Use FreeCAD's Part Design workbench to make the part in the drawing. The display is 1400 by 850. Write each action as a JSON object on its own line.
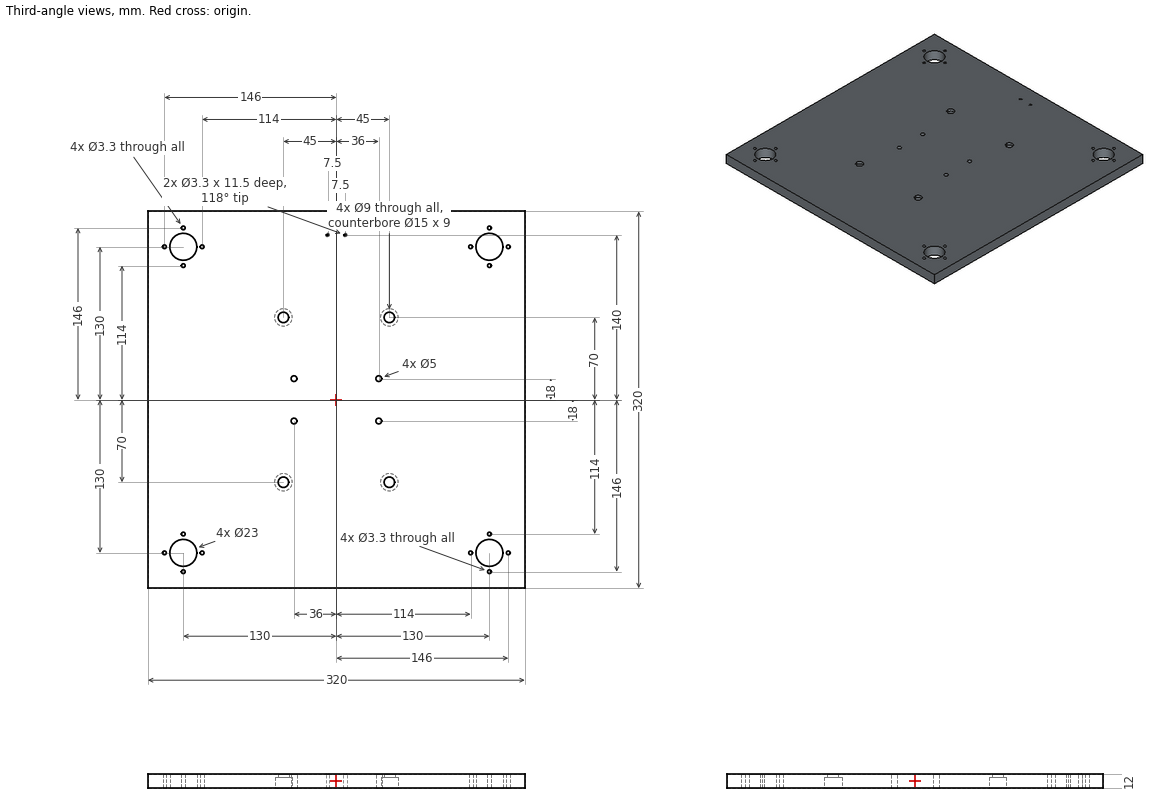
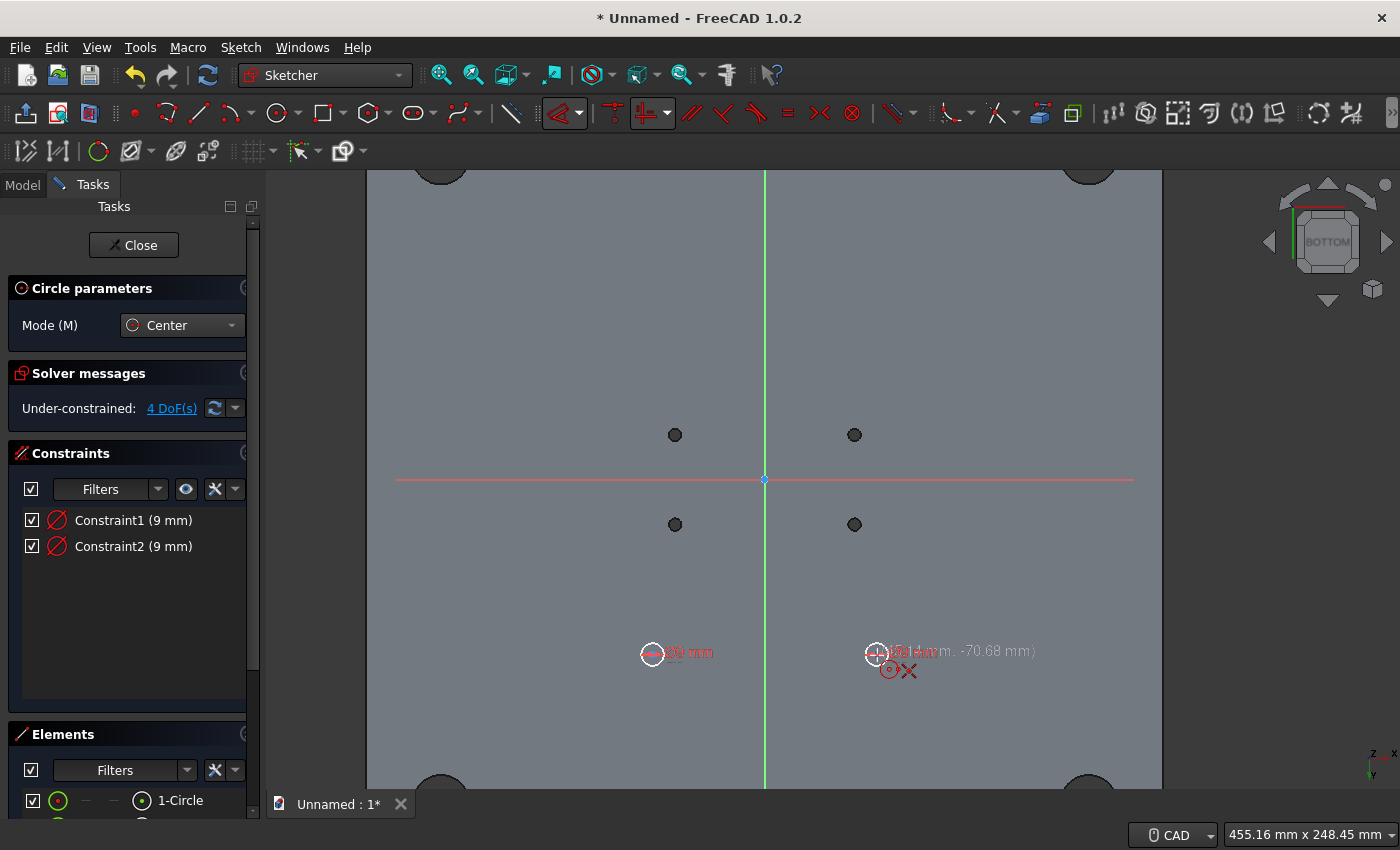
{"action": "scroll", "coordinate": [653, 305], "scroll_direction": "up", "scroll_amount": 4}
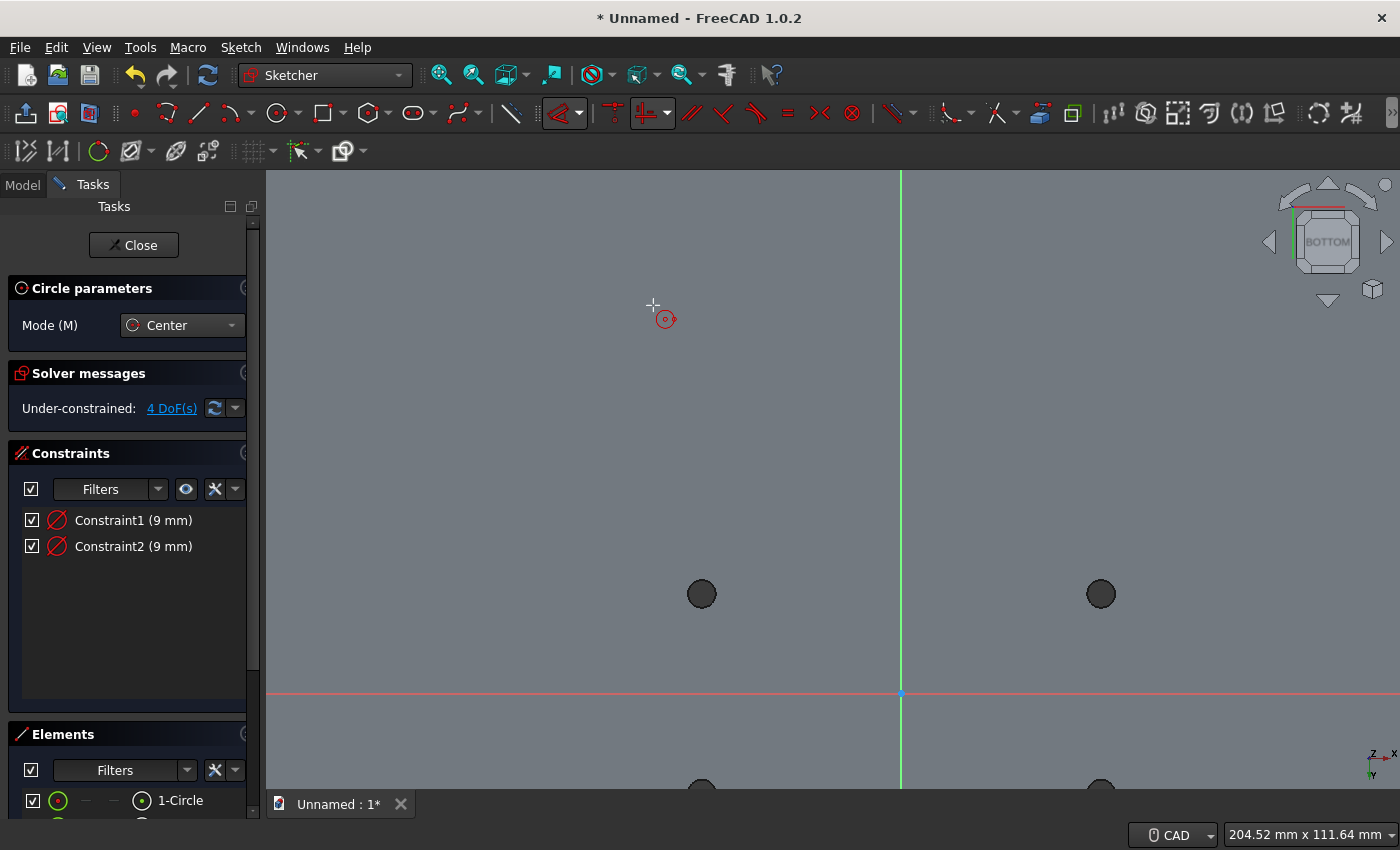
{"action": "left_click", "coordinate": [652, 306]}
{"action": "mouse_move", "coordinate": [670, 288]}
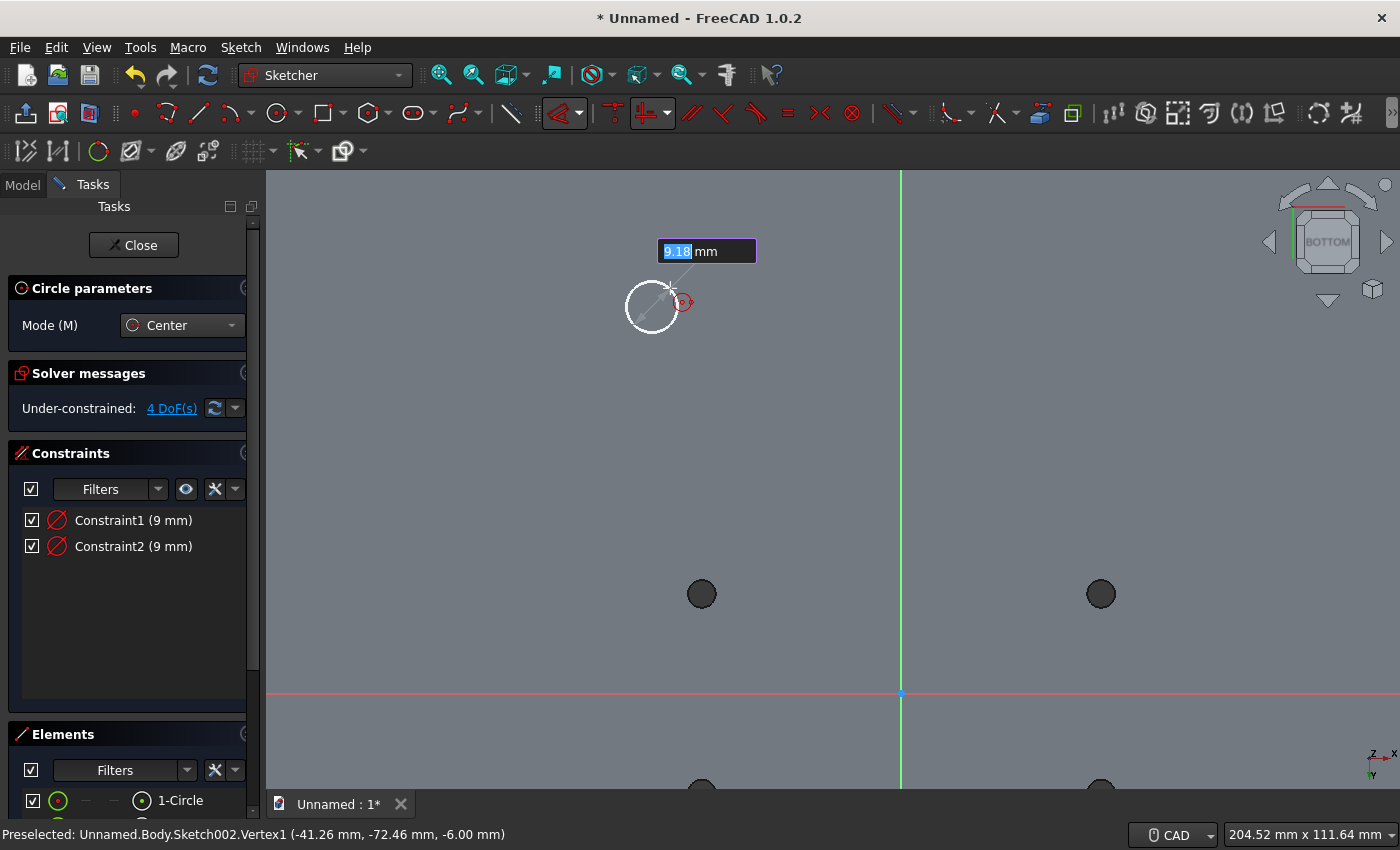
{"action": "type", "text": "9"}
{"action": "key", "text": "Return"}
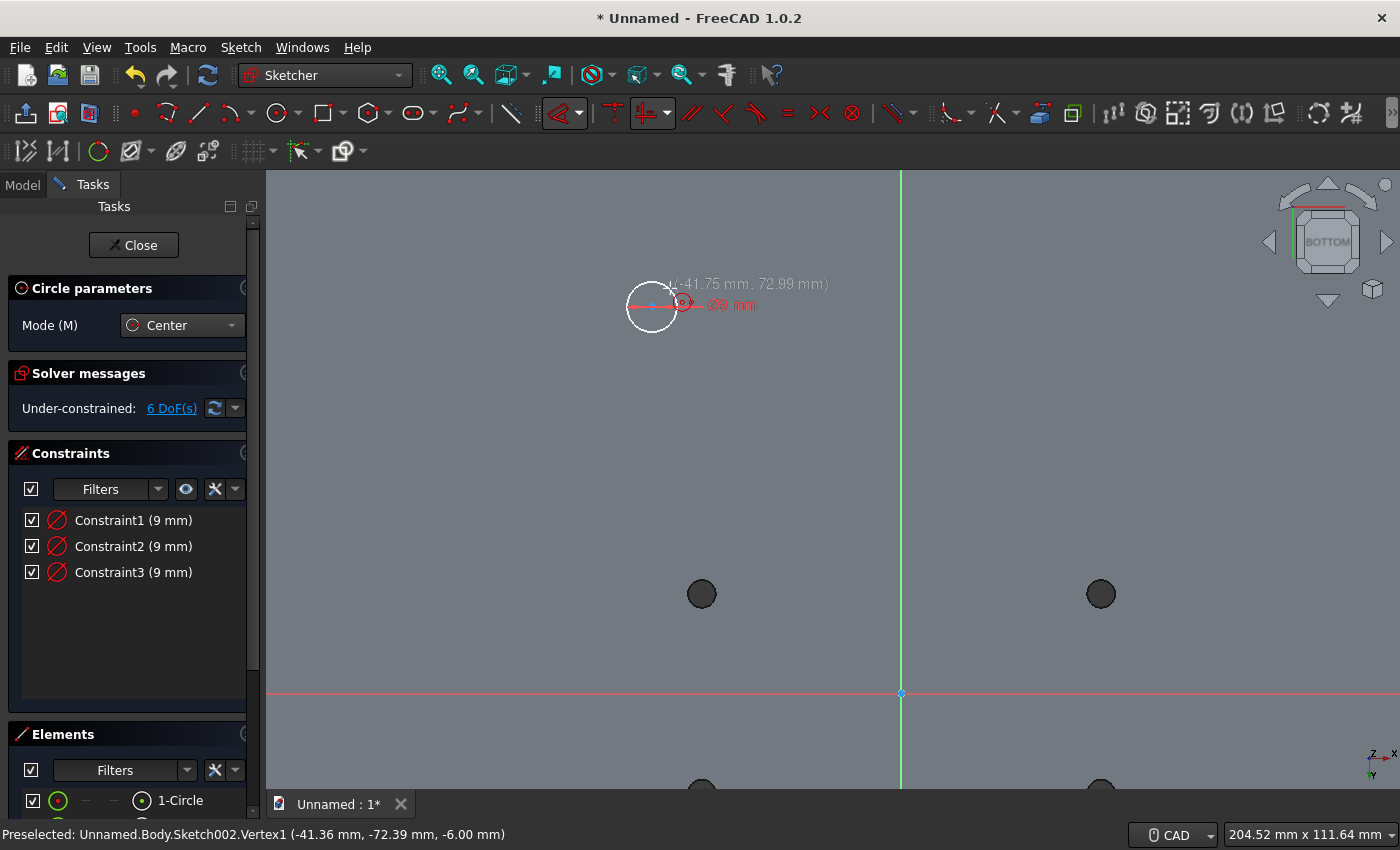
{"action": "left_click", "coordinate": [1151, 306]}
{"action": "mouse_move", "coordinate": [1169, 288]}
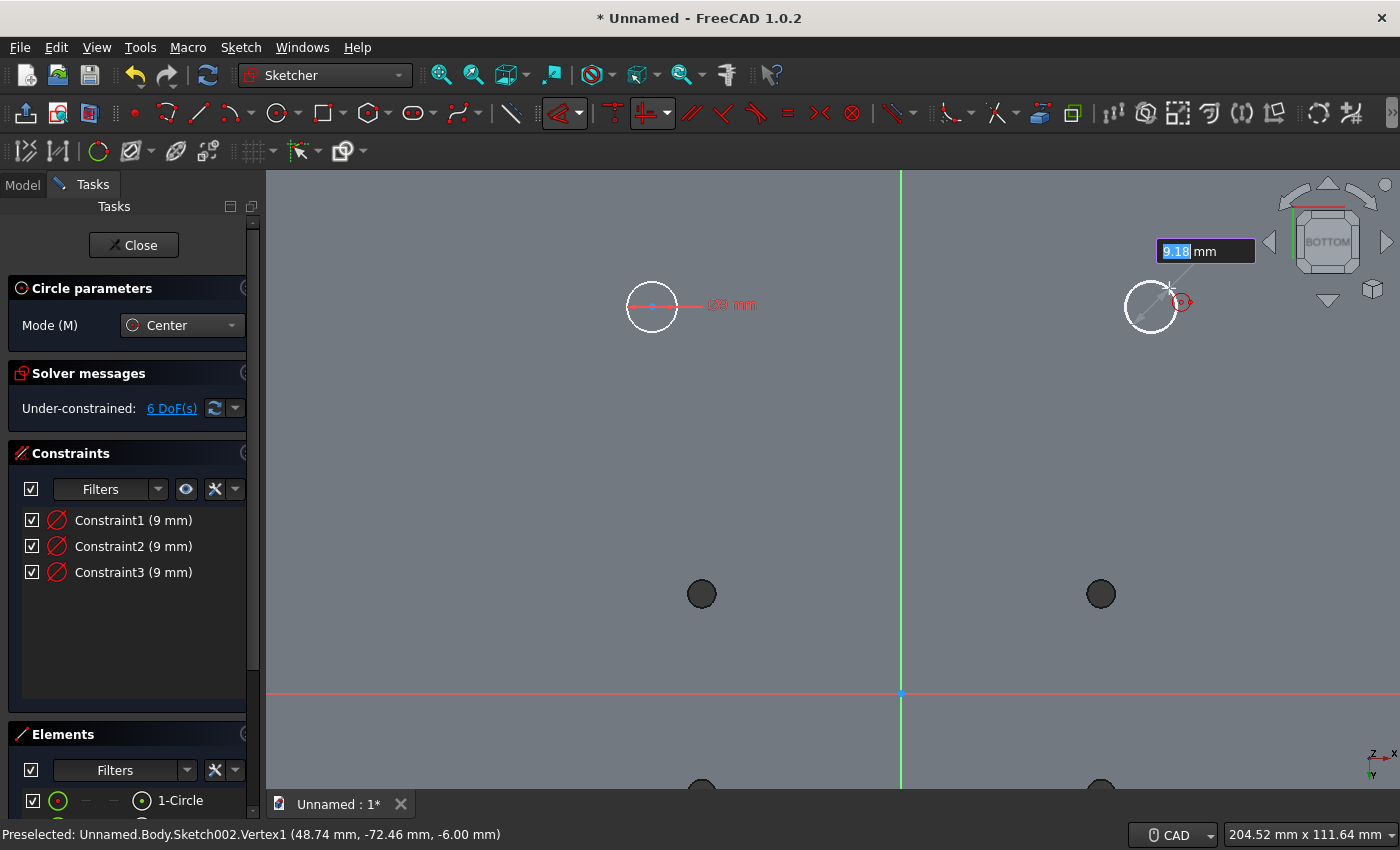
{"action": "type", "text": "9"}
{"action": "key", "text": "Return"}
{"action": "key", "text": "Escape"}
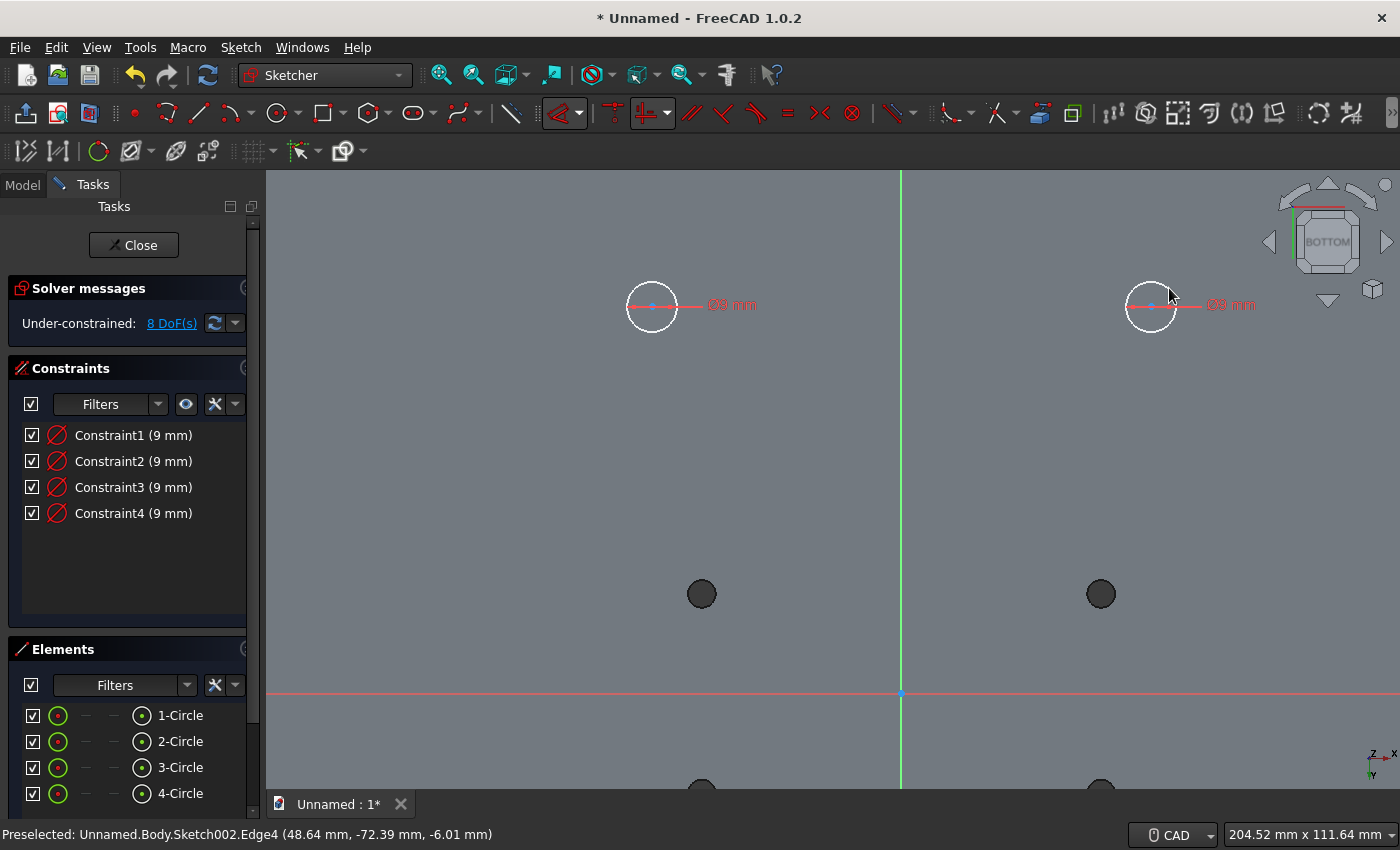
{"action": "scroll", "coordinate": [653, 305], "scroll_direction": "down", "scroll_amount": 4}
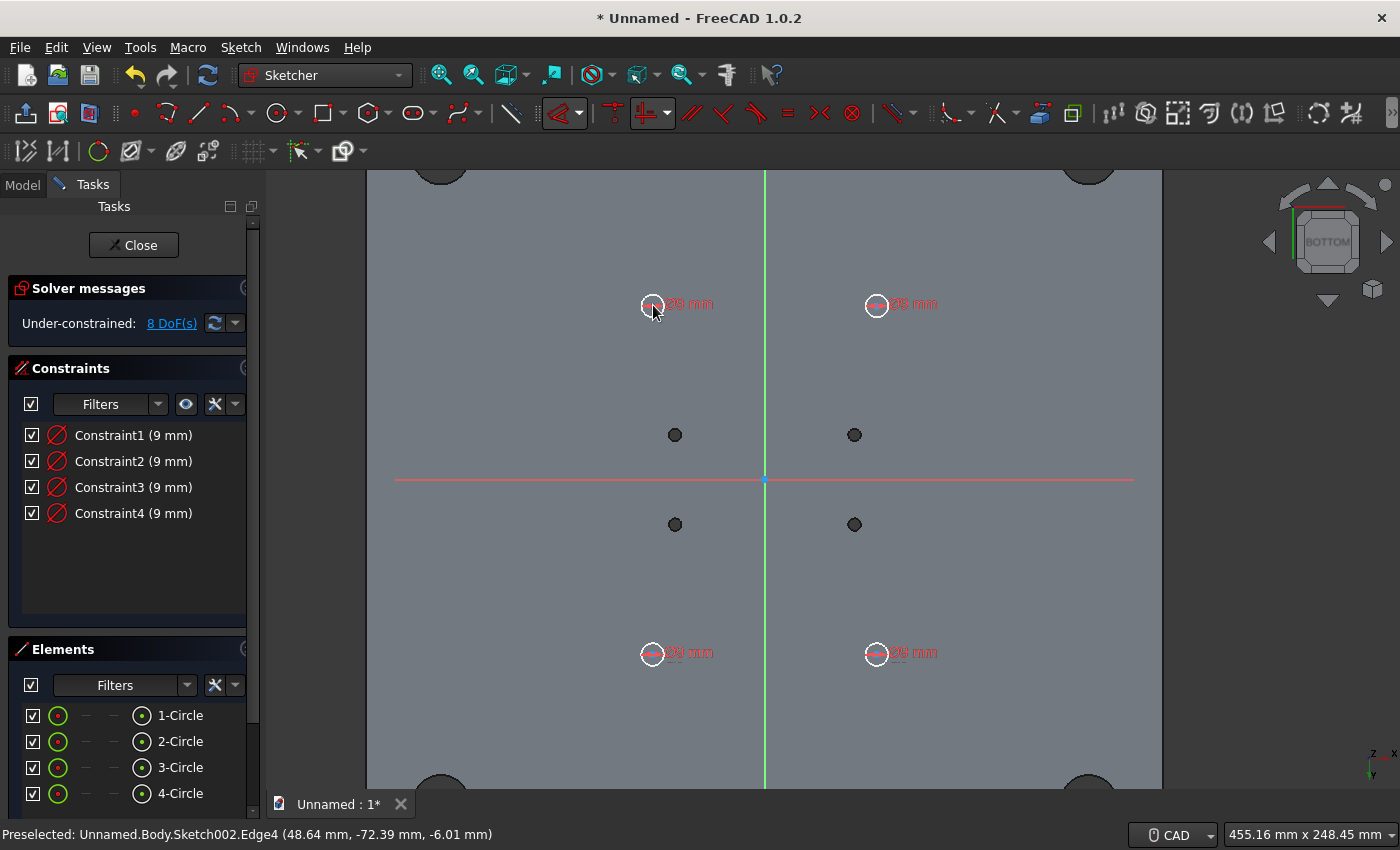
{"action": "left_click", "coordinate": [877, 655]}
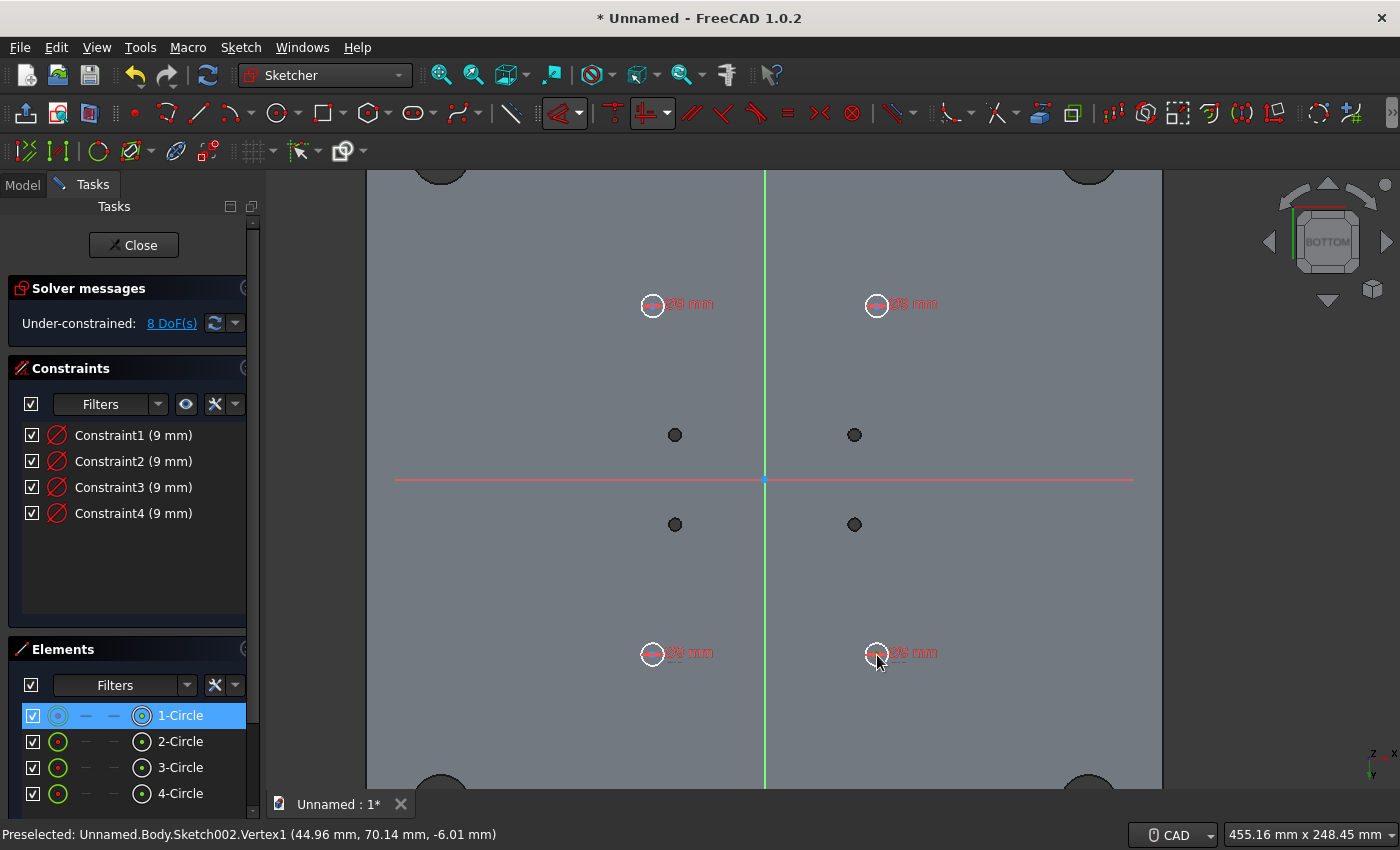
{"action": "left_click", "coordinate": [653, 655]}